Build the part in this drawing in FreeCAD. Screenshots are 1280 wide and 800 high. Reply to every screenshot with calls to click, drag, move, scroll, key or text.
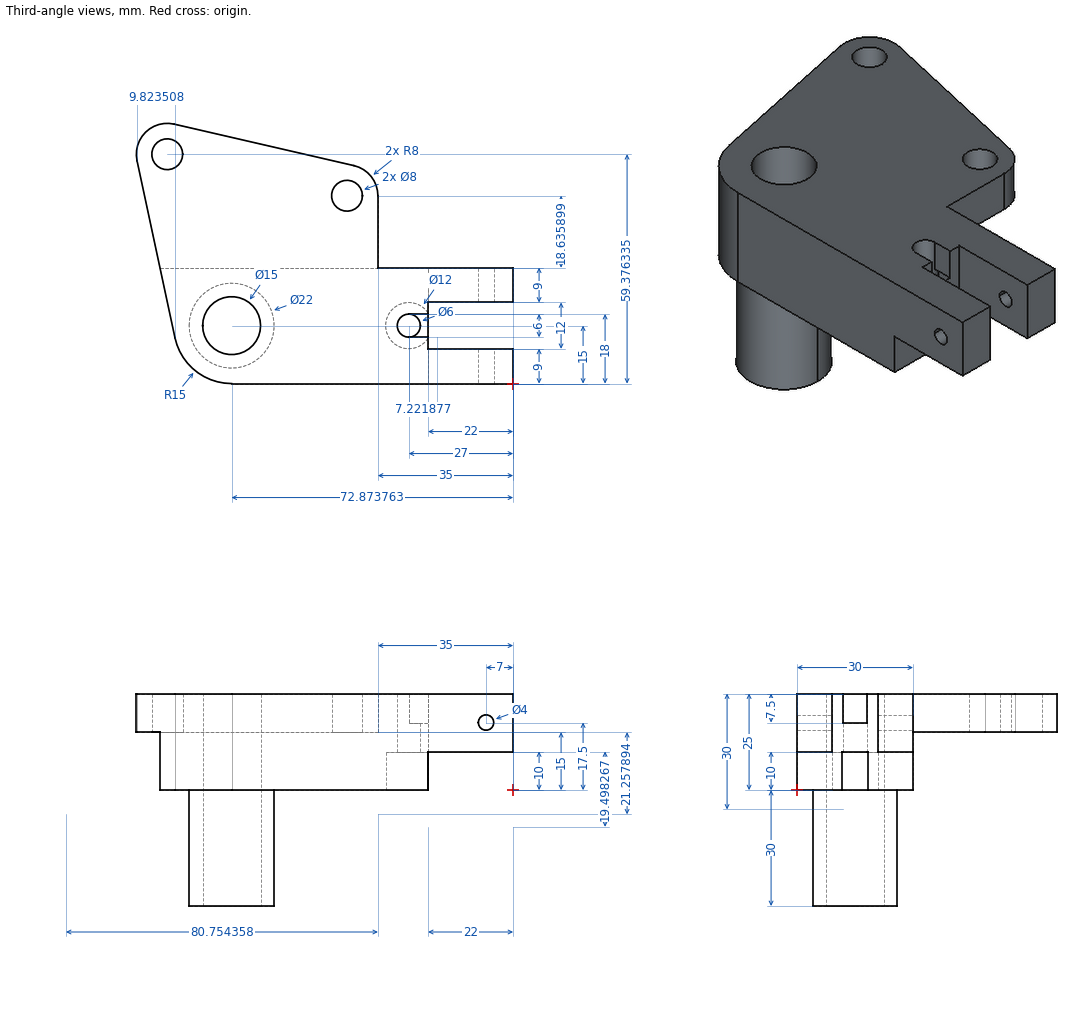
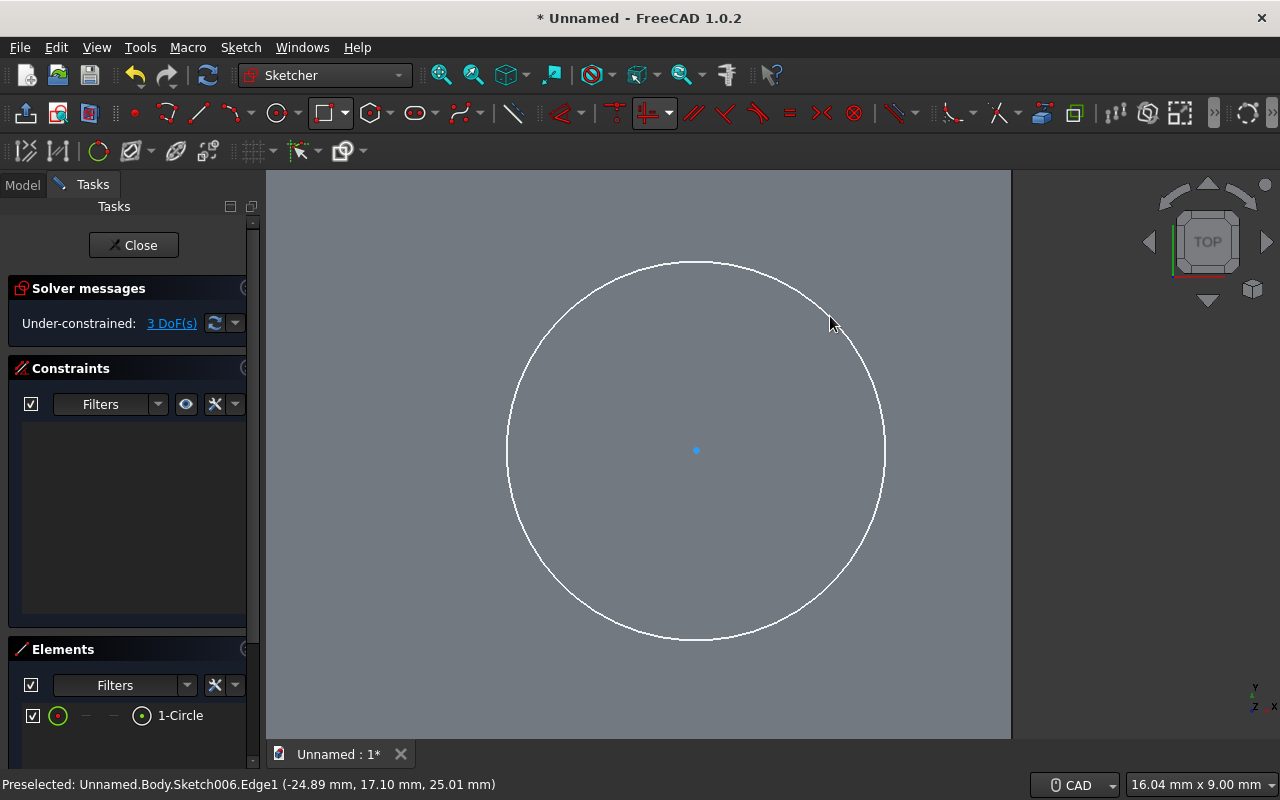
click(560, 114)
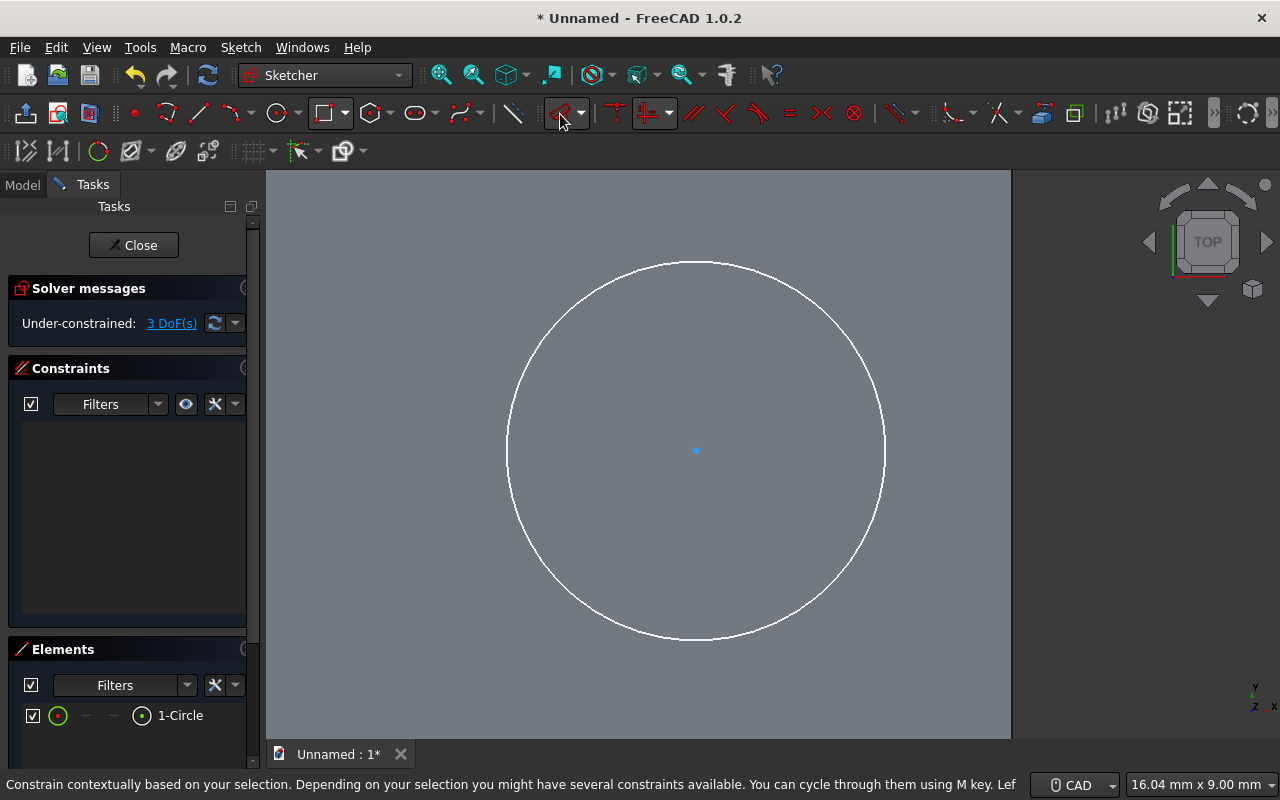
click(830, 317)
click(853, 294)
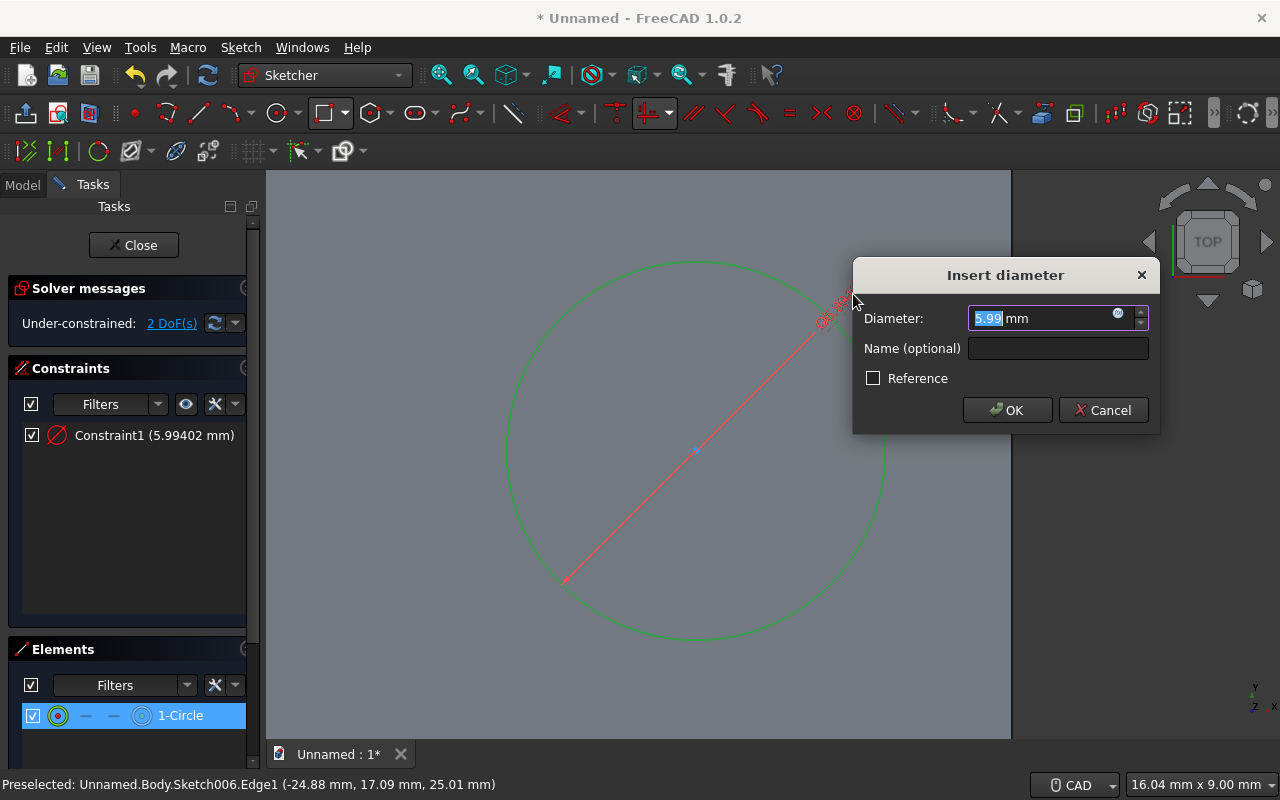
text(6)
key(Return)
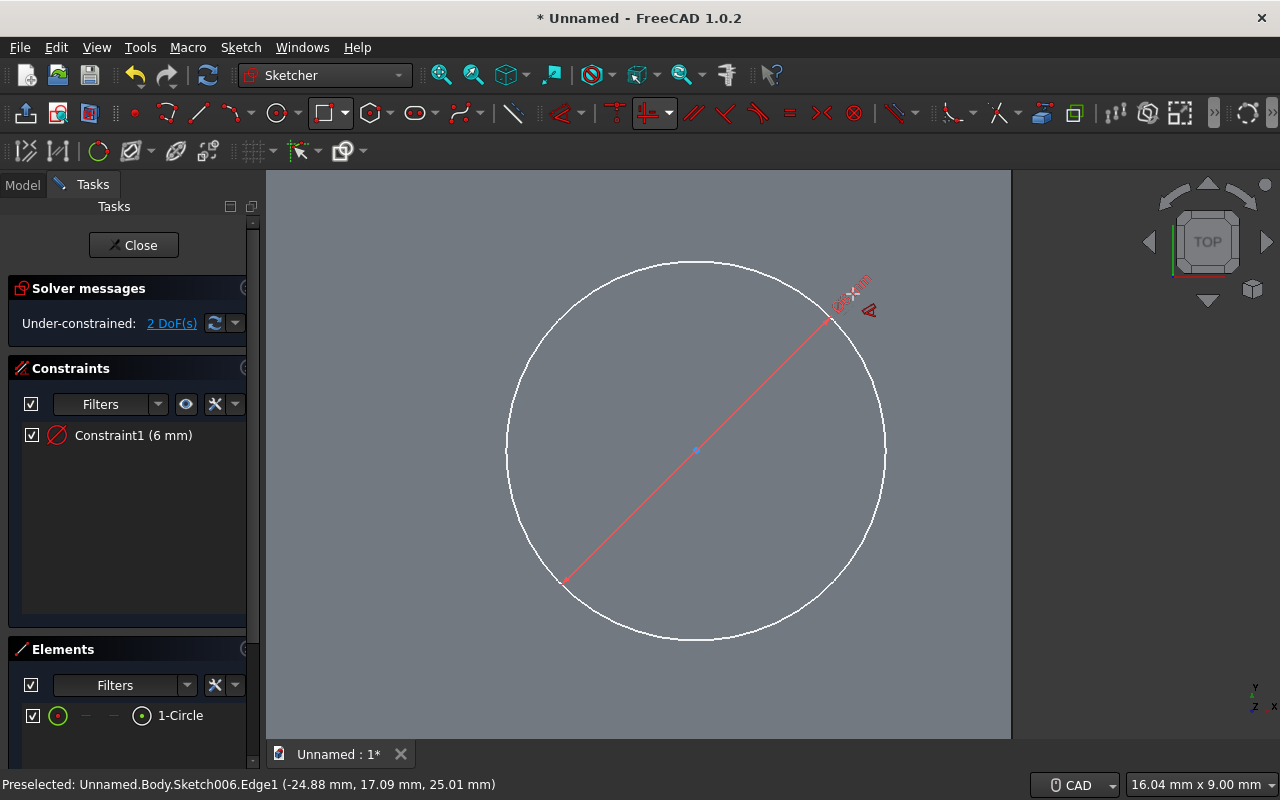
click(696, 451)
click(906, 417)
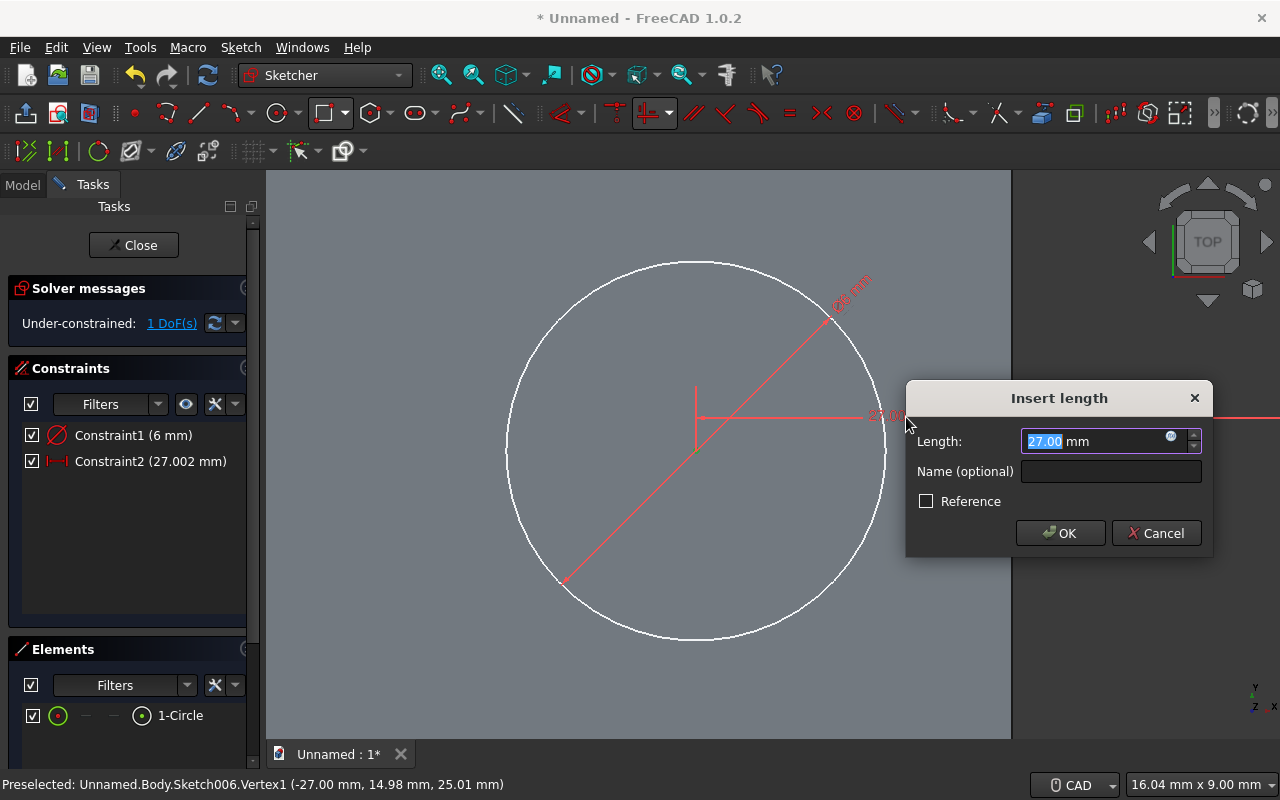
text(27)
key(Return)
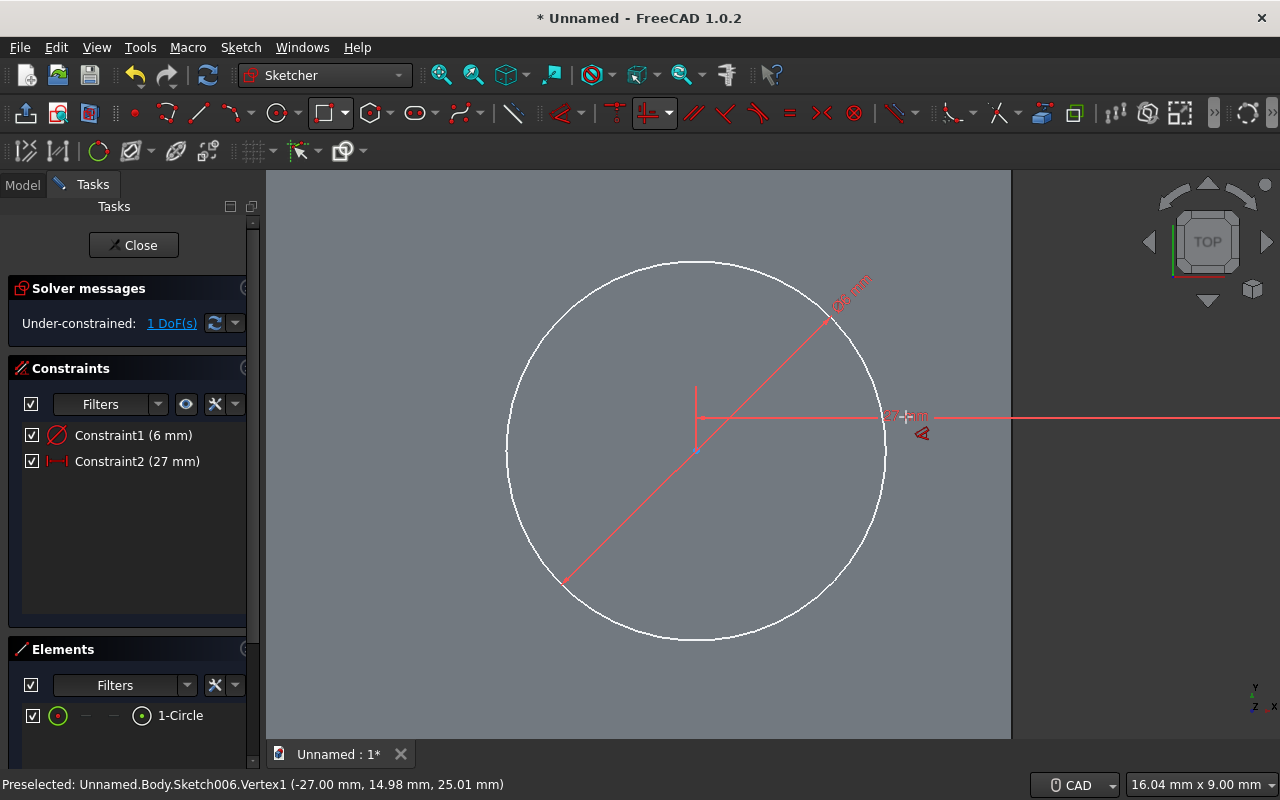
click(696, 451)
click(662, 581)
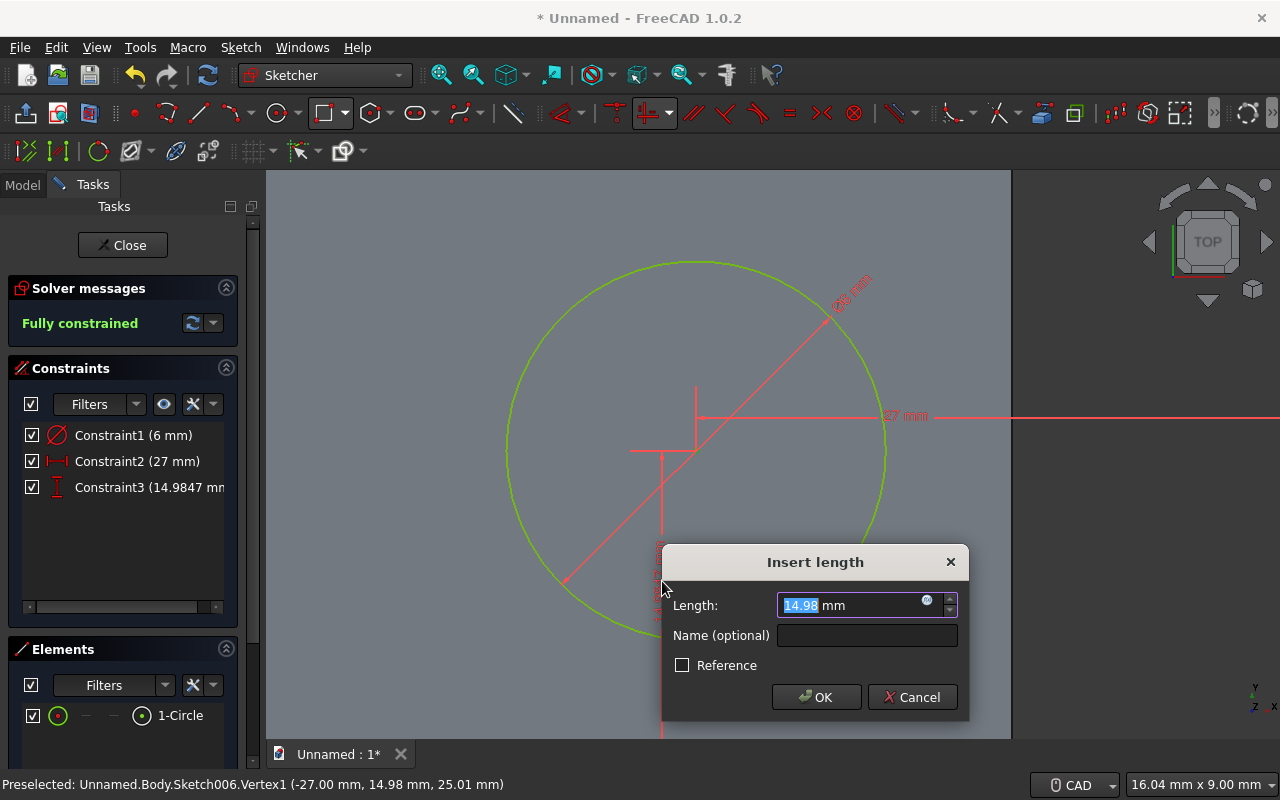
text(15)
key(Return)
key(Escape)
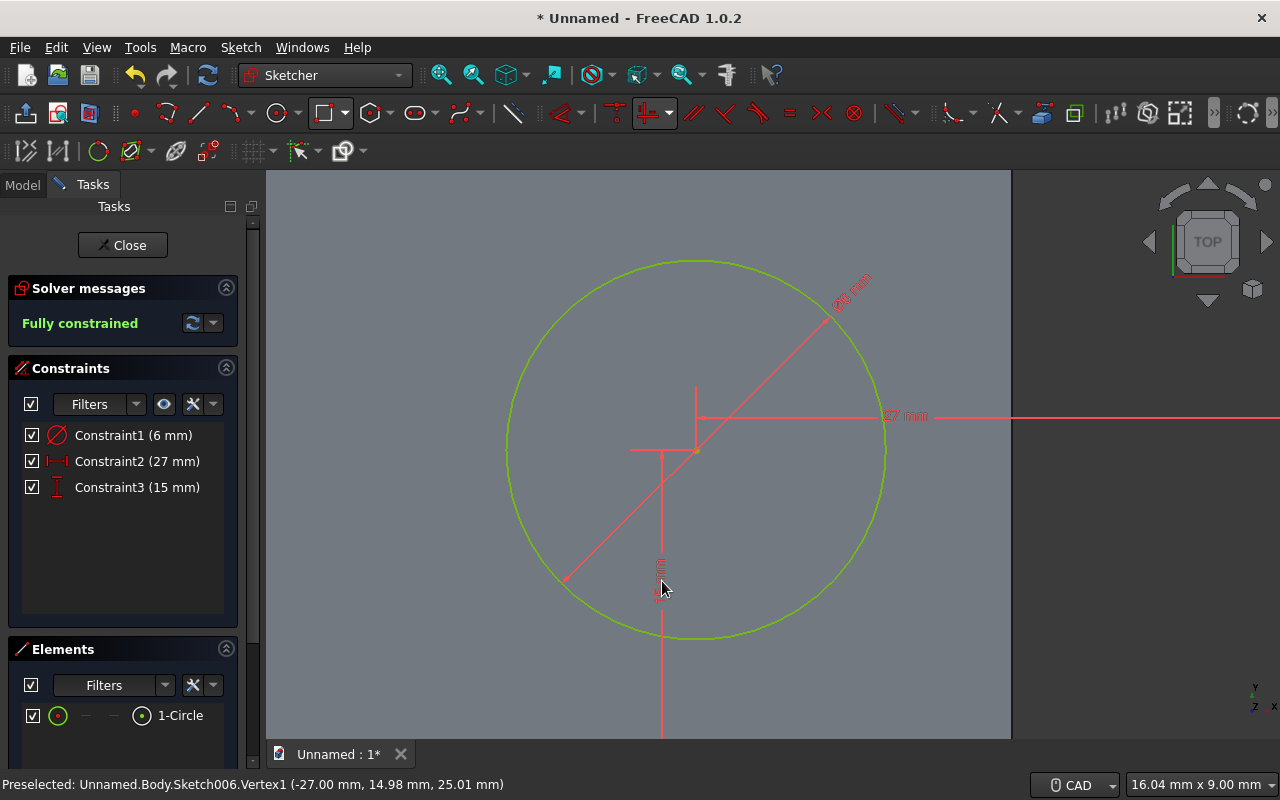
click(123, 245)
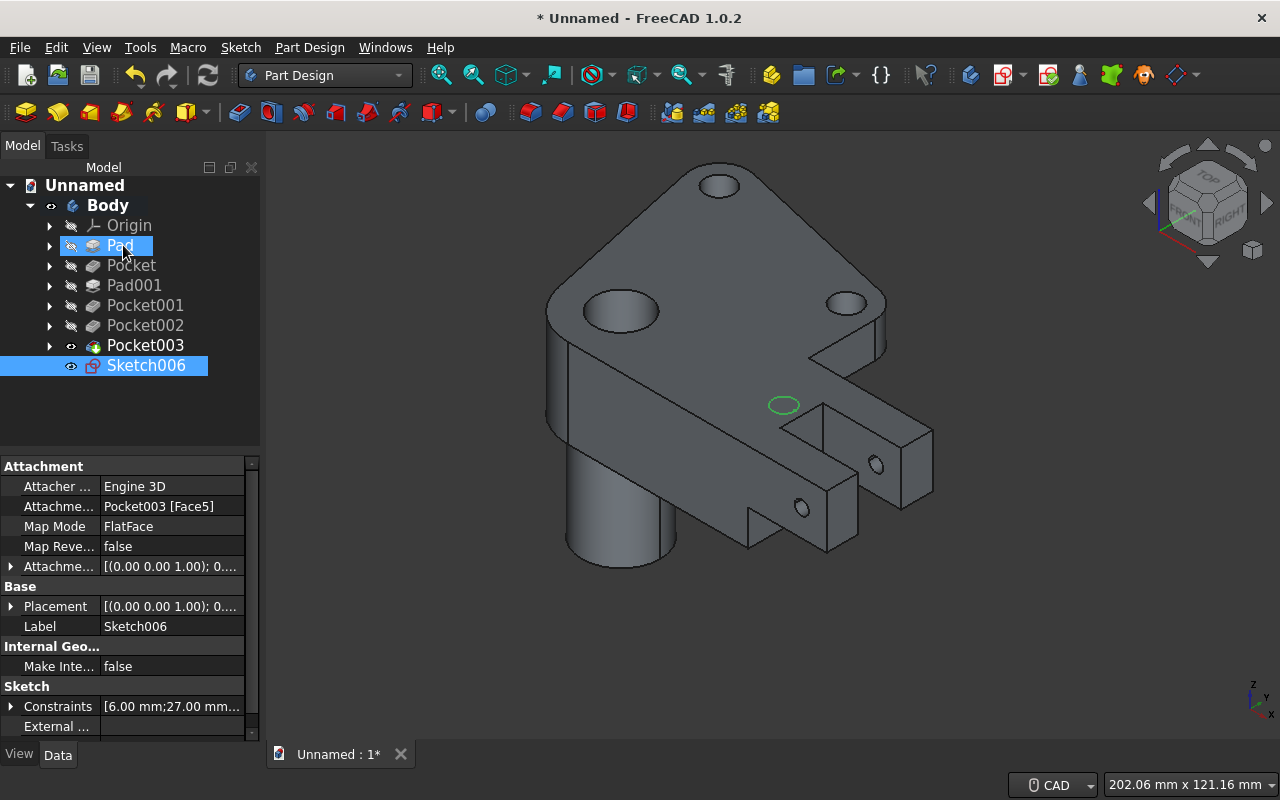
click(240, 112)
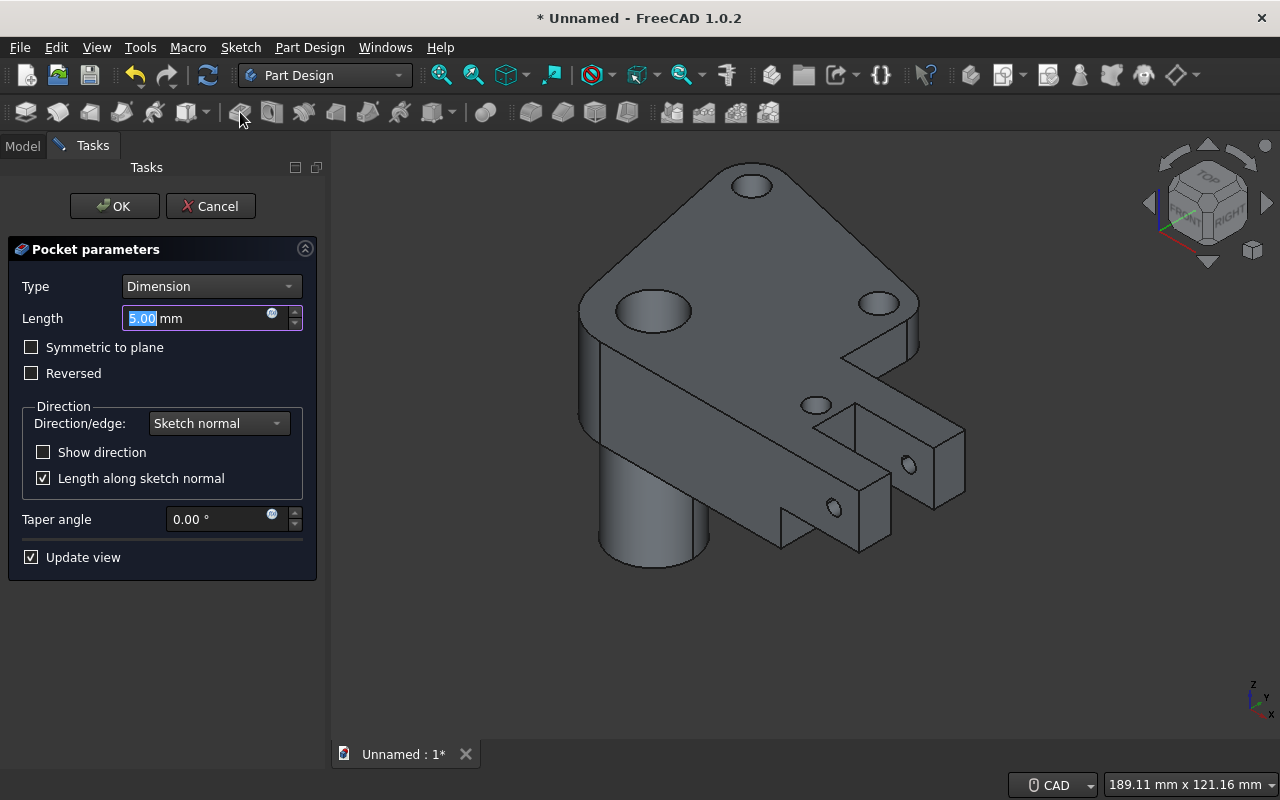
text(30)
key(Tab)